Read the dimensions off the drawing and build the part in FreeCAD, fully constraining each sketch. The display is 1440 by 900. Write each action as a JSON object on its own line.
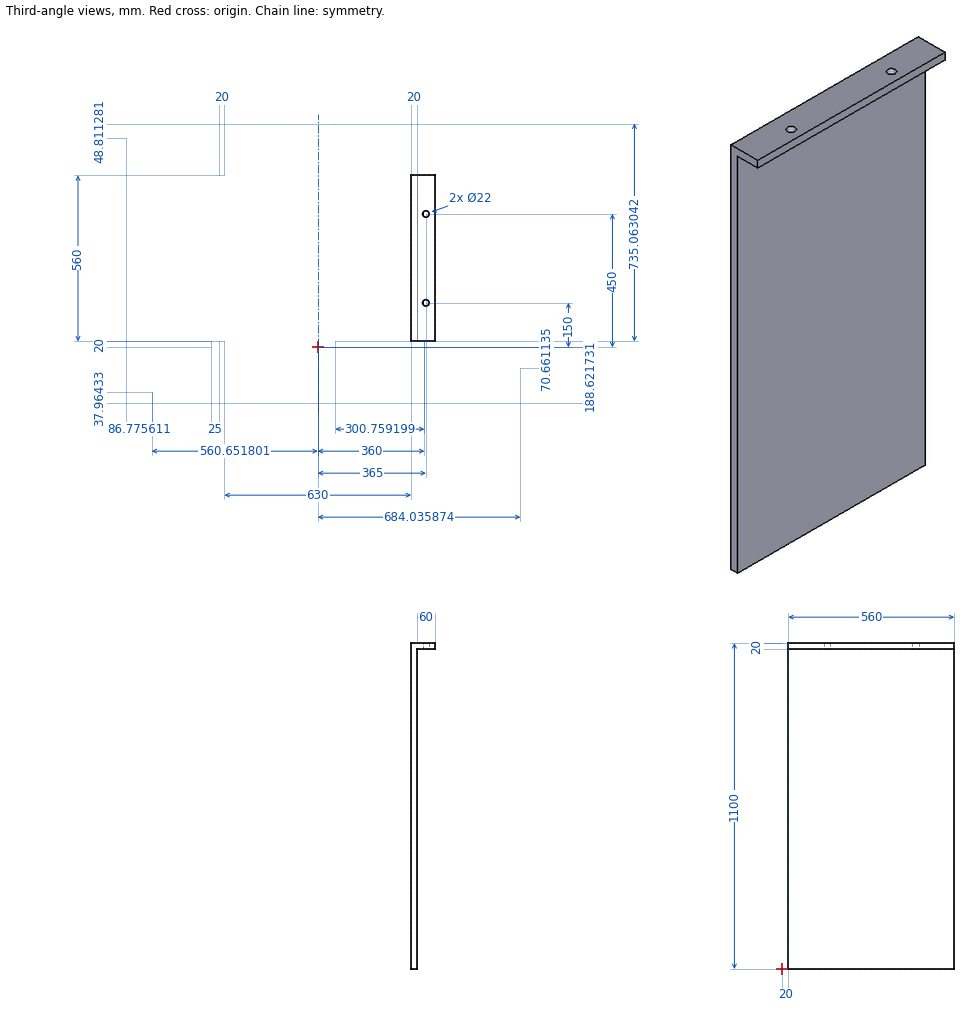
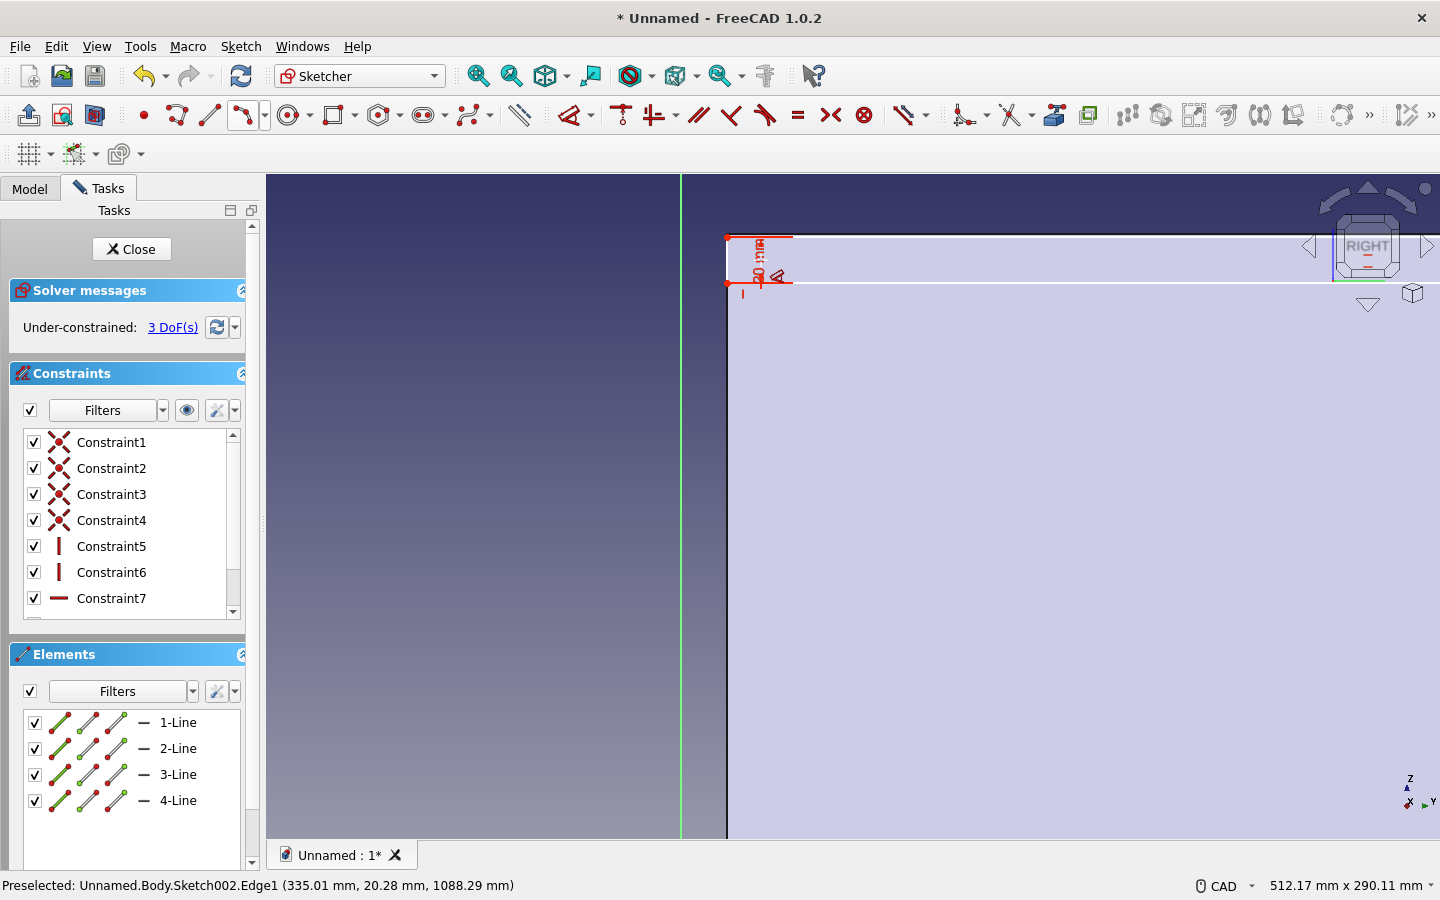
{"action": "scroll", "coordinate": [673, 311], "scroll_direction": "down", "scroll_amount": 9}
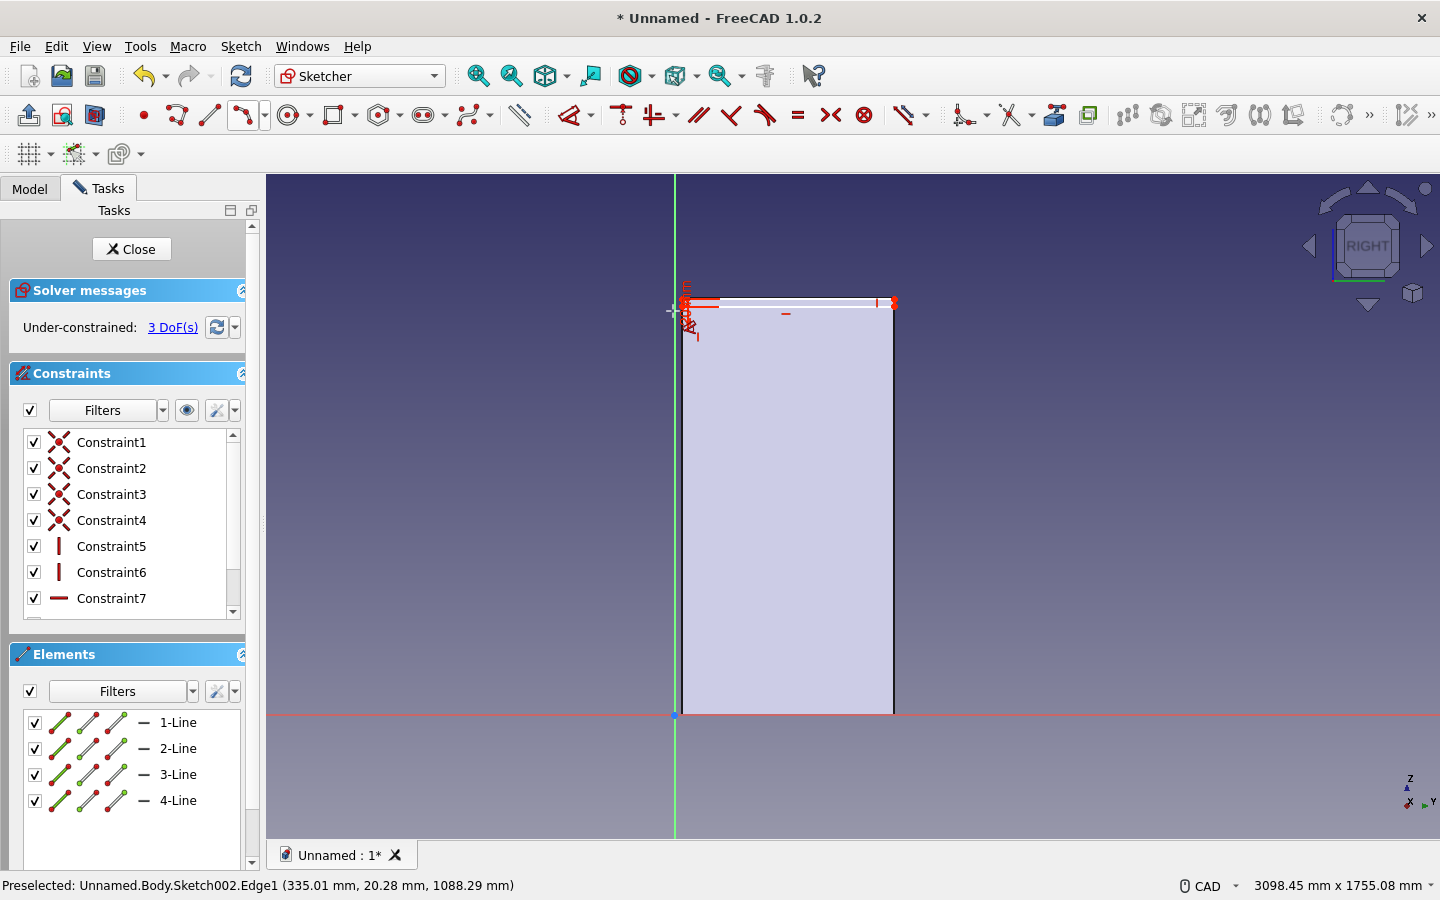
{"action": "scroll", "coordinate": [746, 307], "scroll_direction": "up", "scroll_amount": 3}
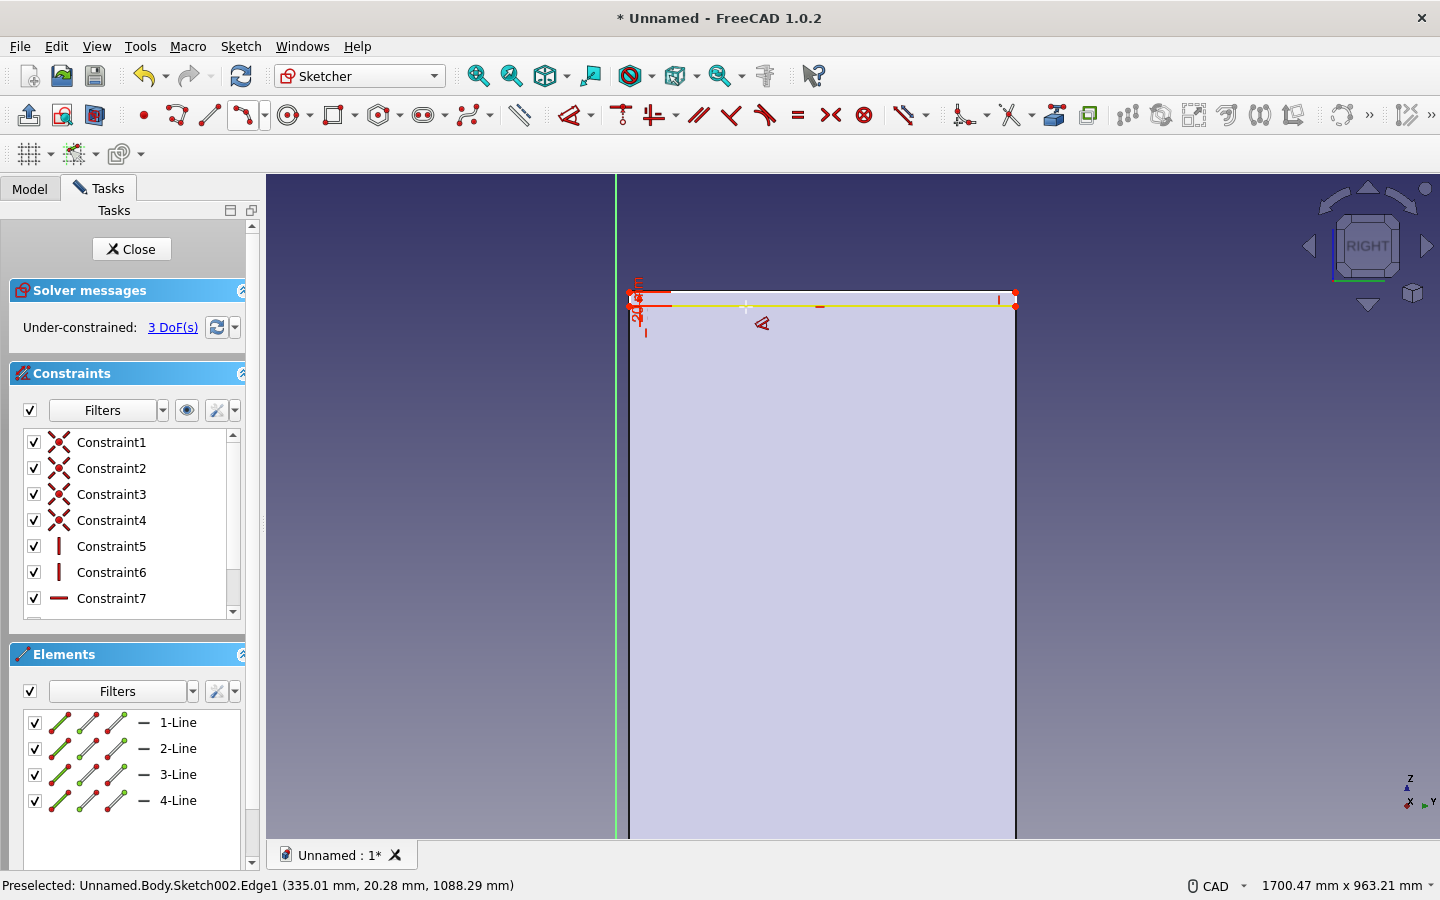
{"action": "left_click", "coordinate": [745, 306]}
{"action": "left_click", "coordinate": [823, 272]}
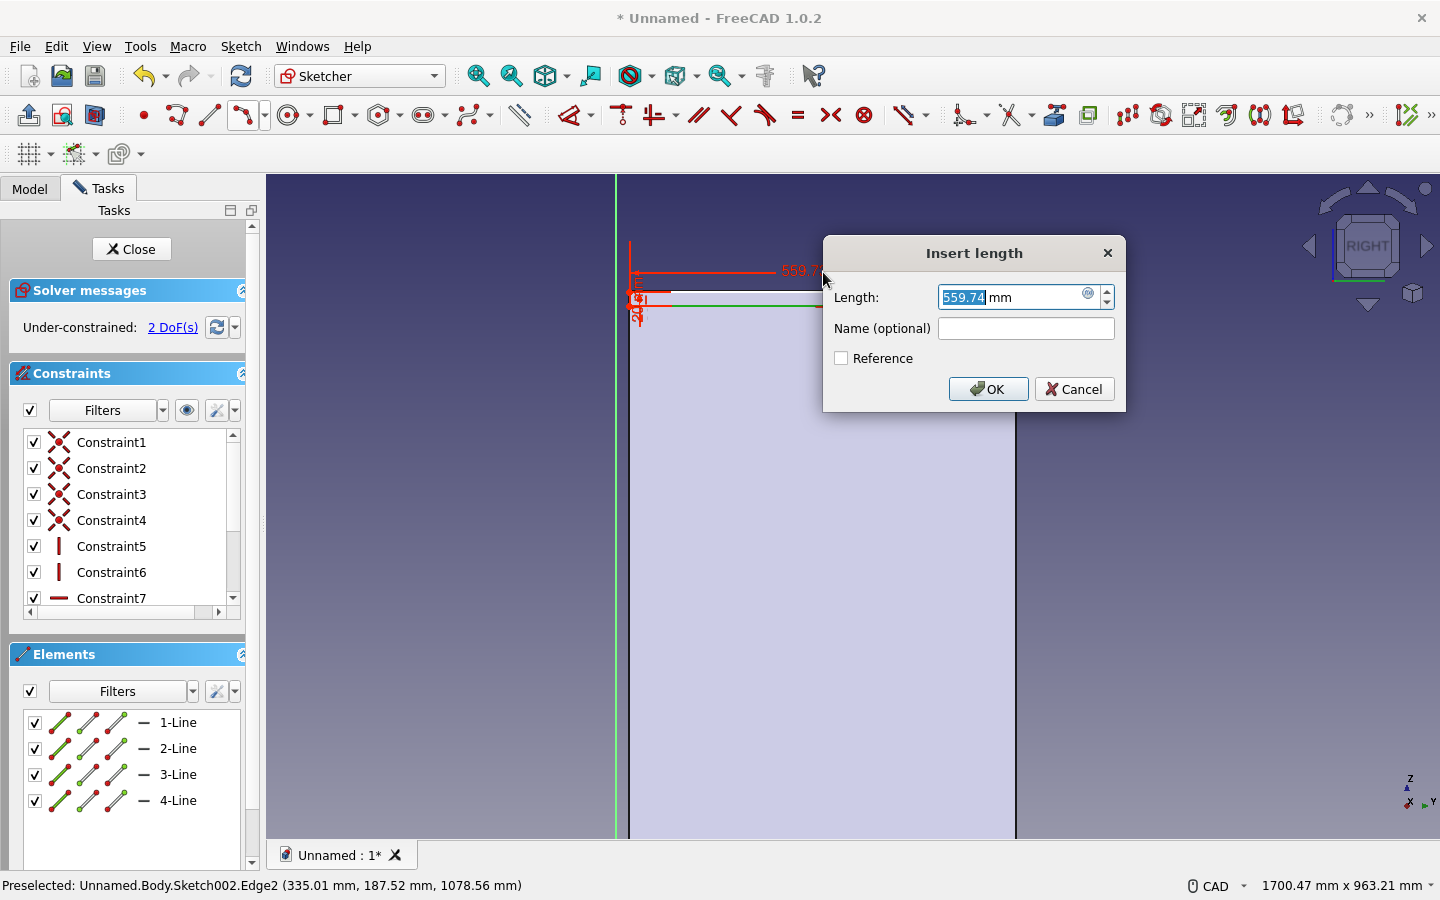
{"action": "type", "text": "560"}
{"action": "key", "text": "Return"}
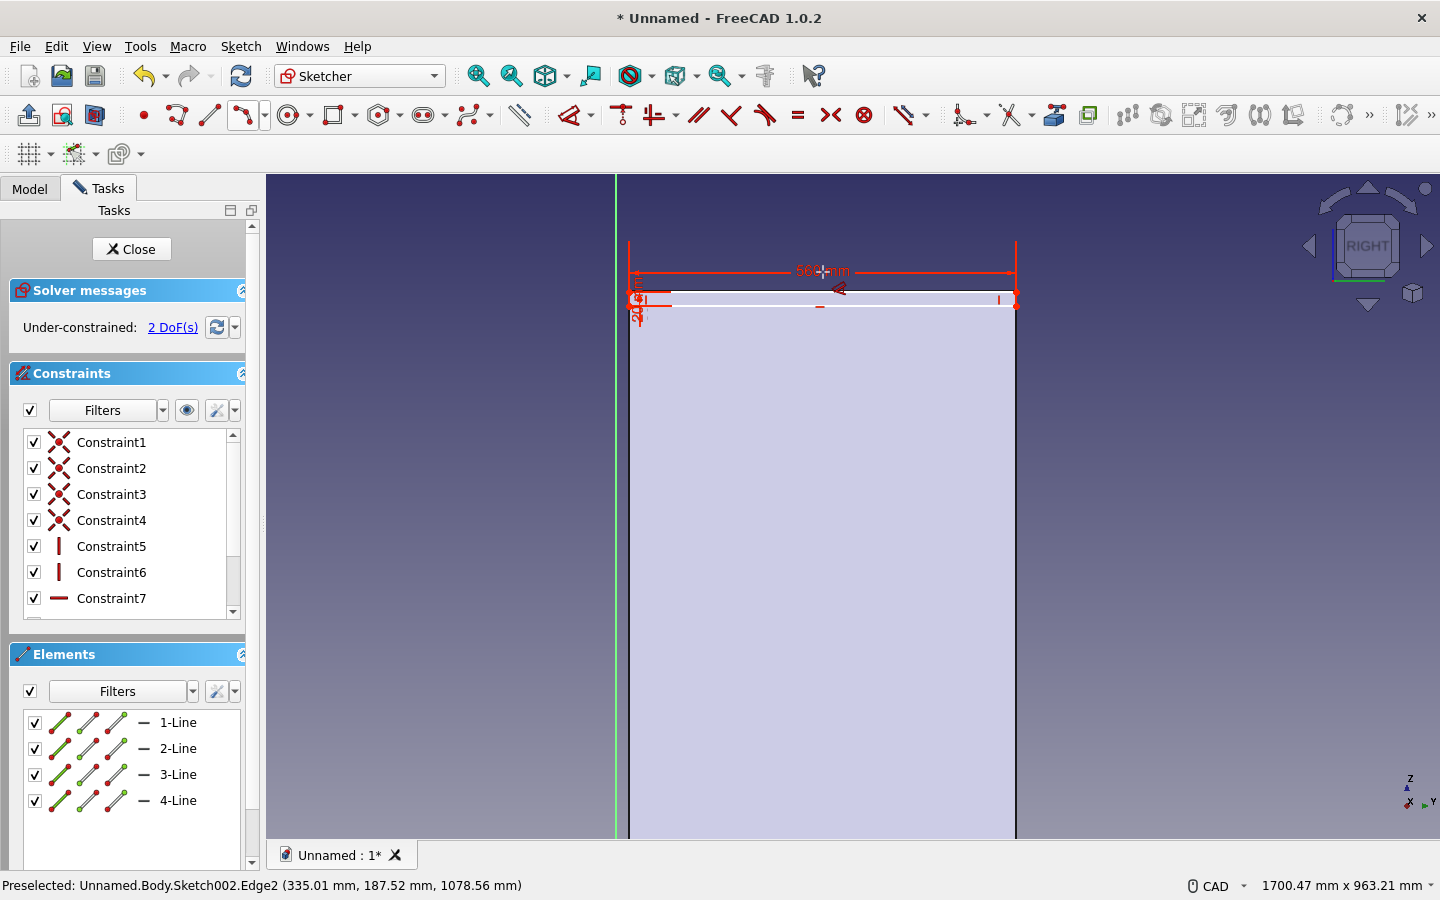
{"action": "scroll", "coordinate": [629, 292], "scroll_direction": "up", "scroll_amount": 6}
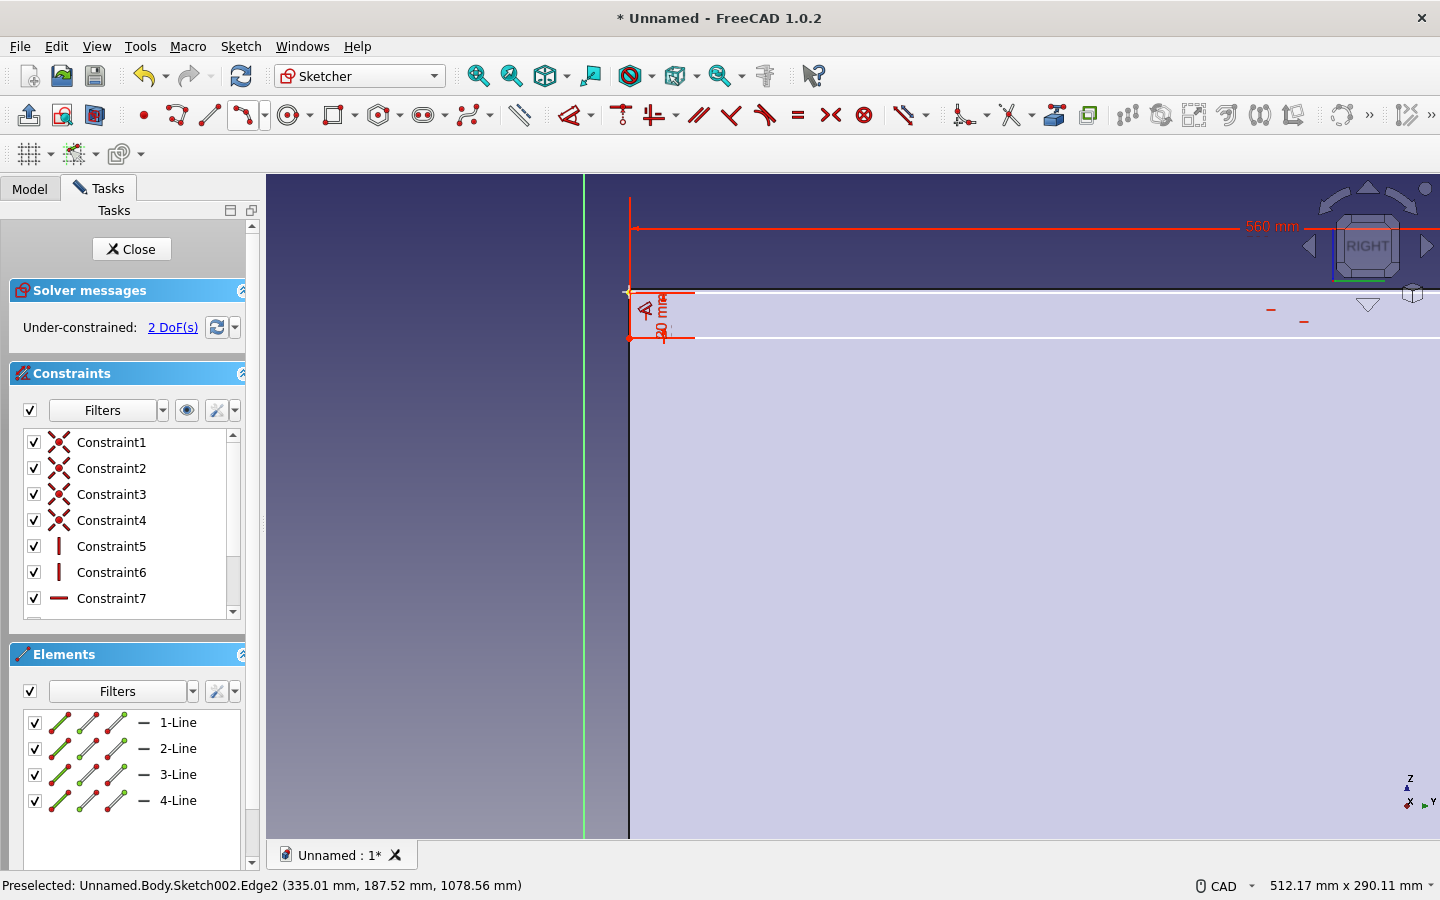
{"action": "left_click", "coordinate": [630, 293]}
{"action": "left_click", "coordinate": [607, 259]}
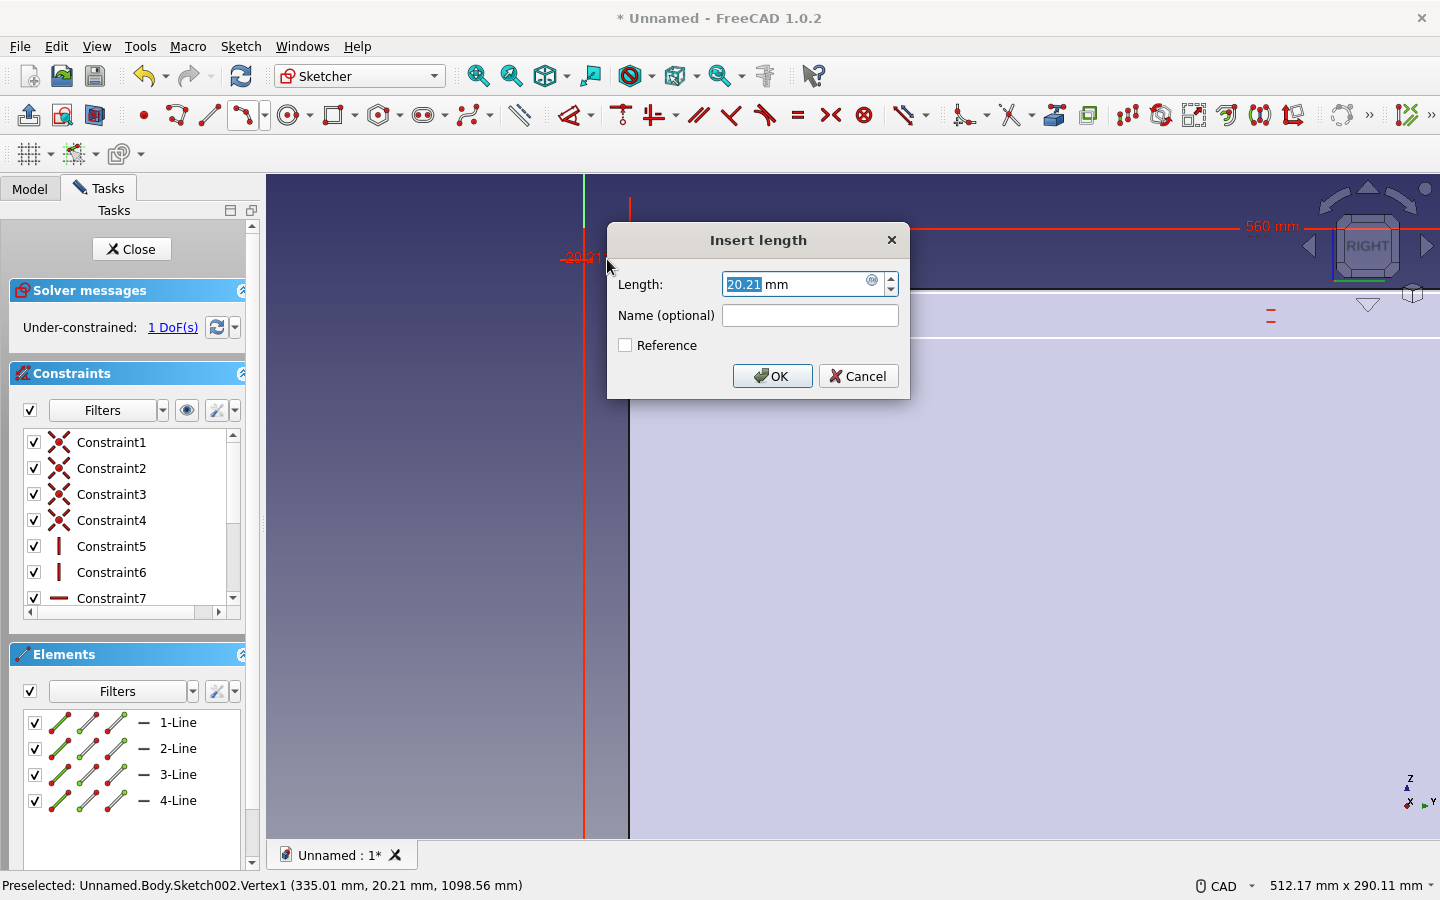
{"action": "type", "text": "20"}
{"action": "key", "text": "Return"}